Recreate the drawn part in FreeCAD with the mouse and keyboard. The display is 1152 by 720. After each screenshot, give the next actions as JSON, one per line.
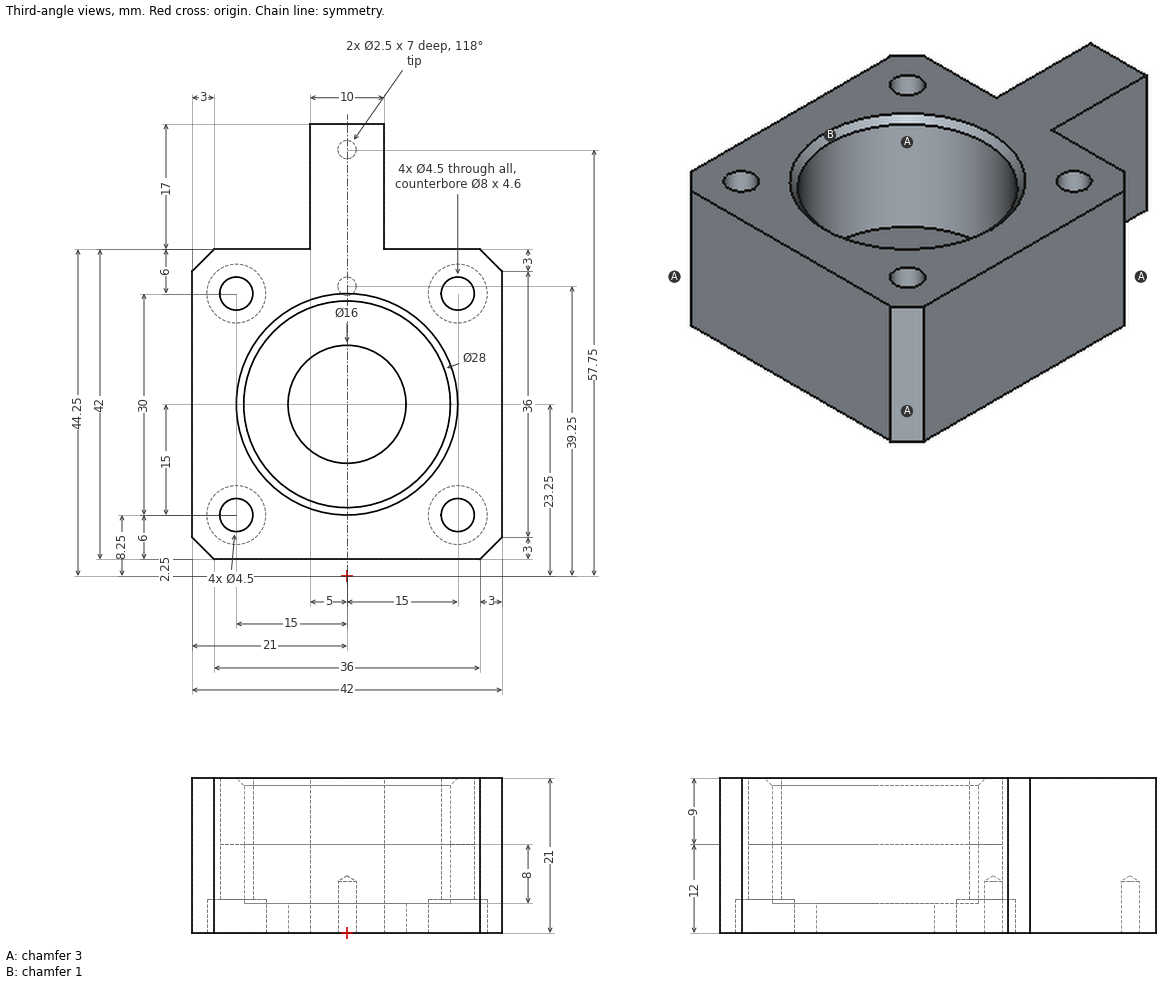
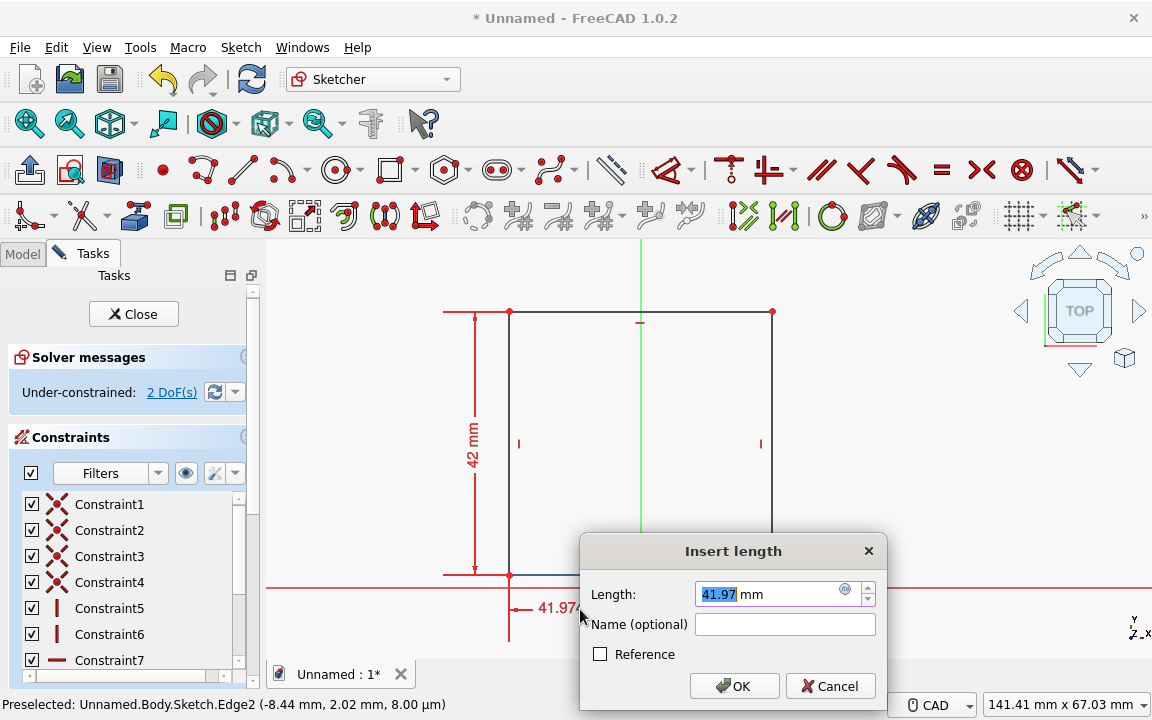
{"action": "type", "text": "42"}
{"action": "key", "text": "Return"}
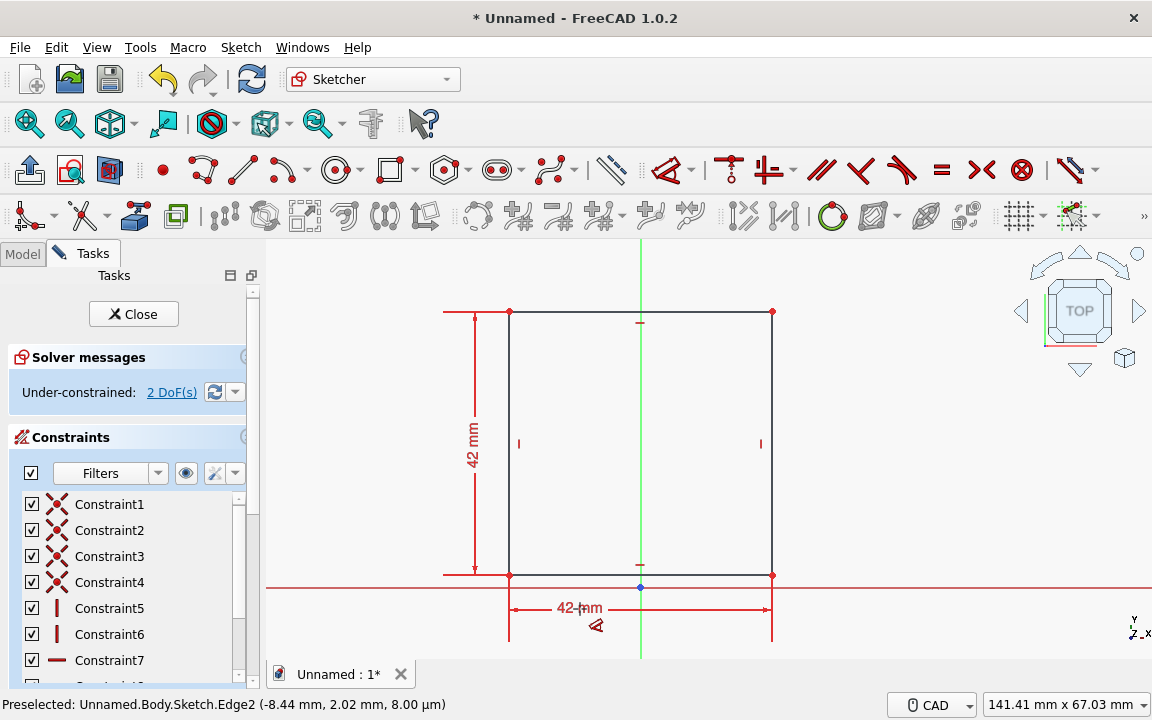
{"action": "left_click", "coordinate": [509, 312]}
{"action": "left_click", "coordinate": [575, 278]}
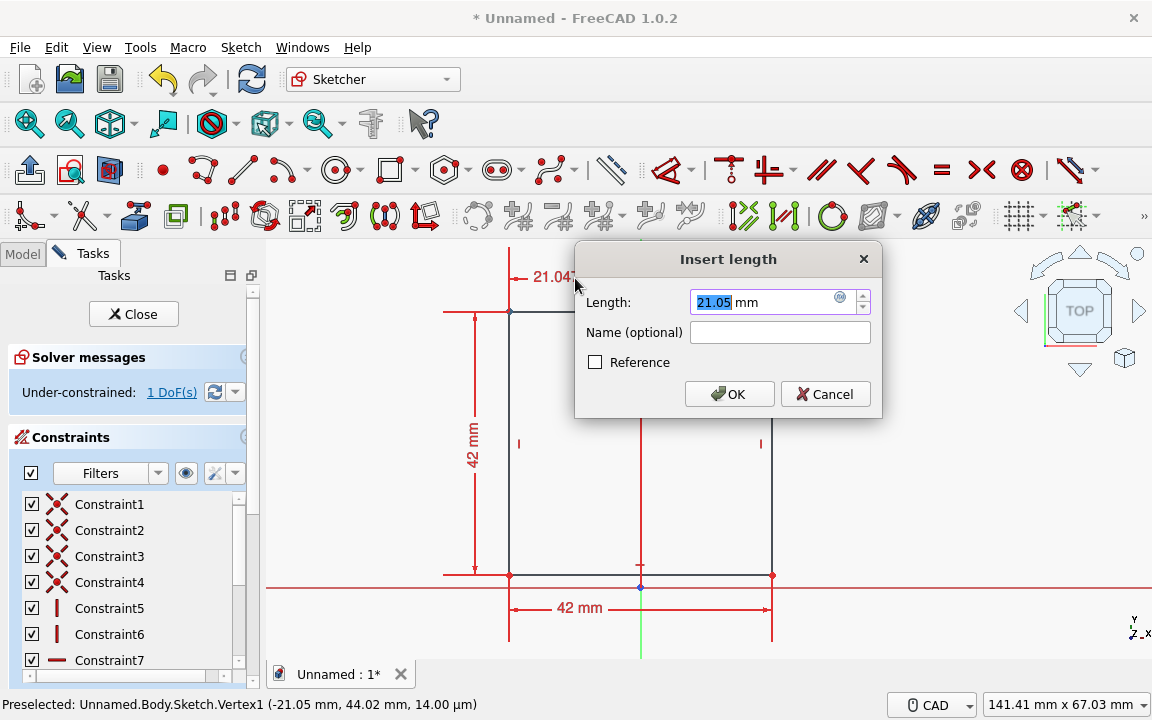
{"action": "type", "text": "21"}
{"action": "key", "text": "Return"}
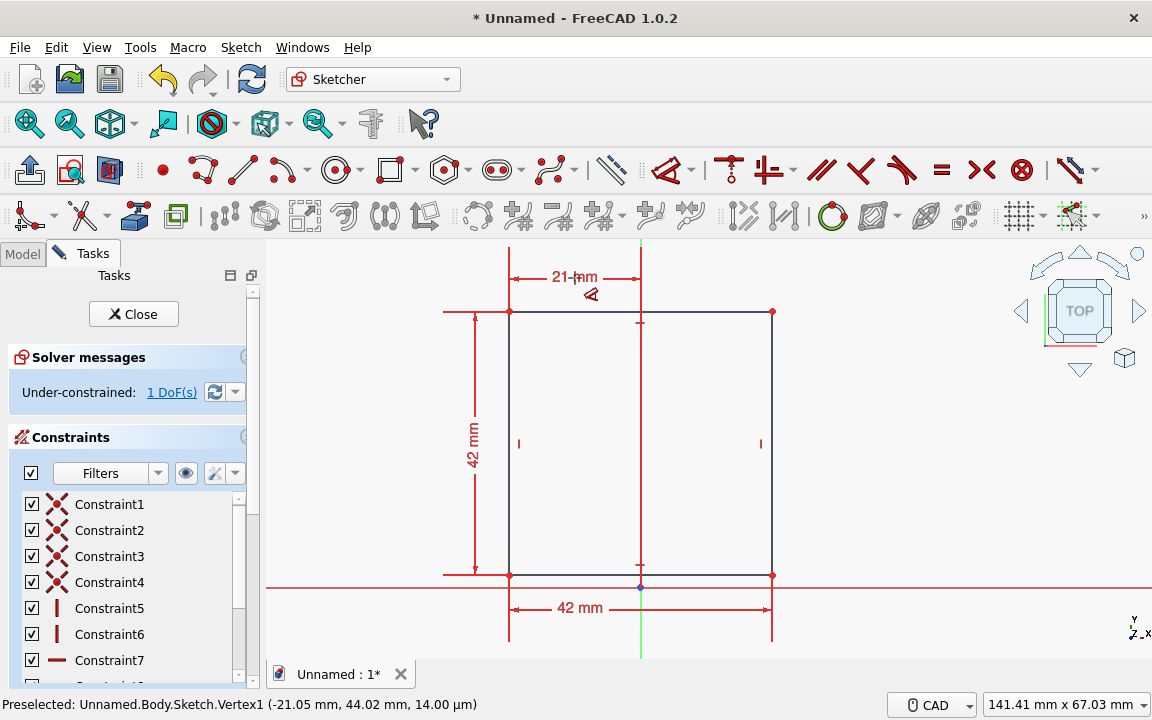
{"action": "scroll", "coordinate": [509, 575], "scroll_direction": "up", "scroll_amount": 6}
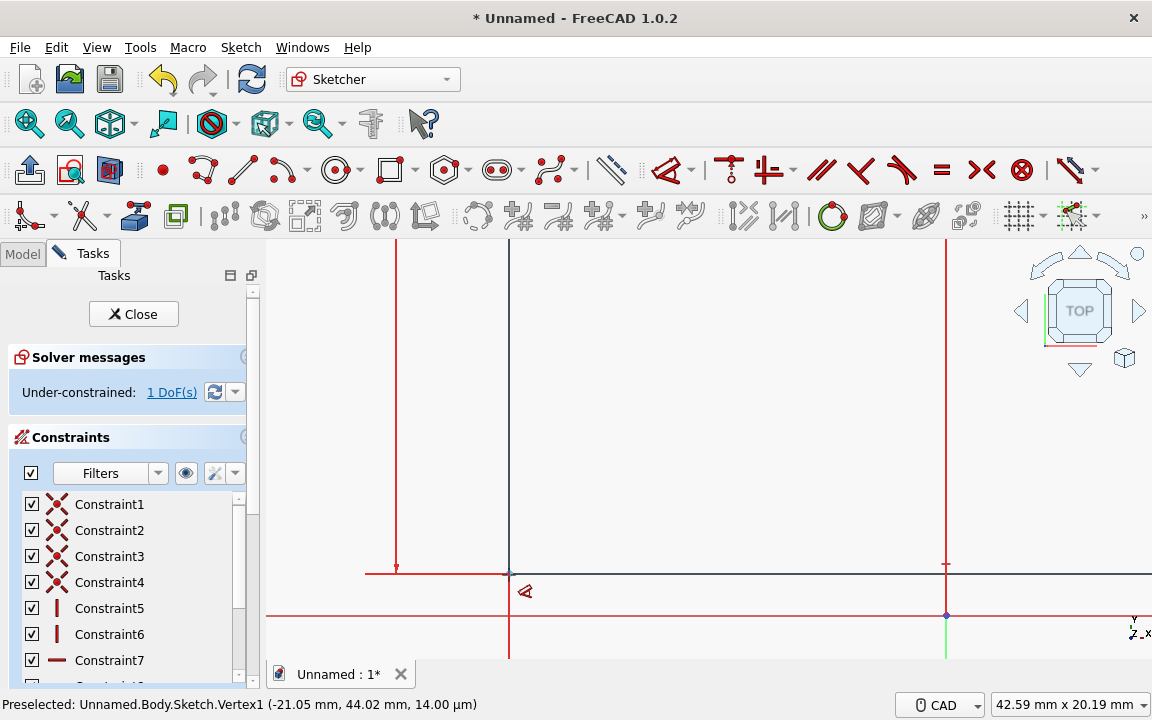
{"action": "left_click", "coordinate": [509, 574]}
{"action": "left_click", "coordinate": [475, 595]}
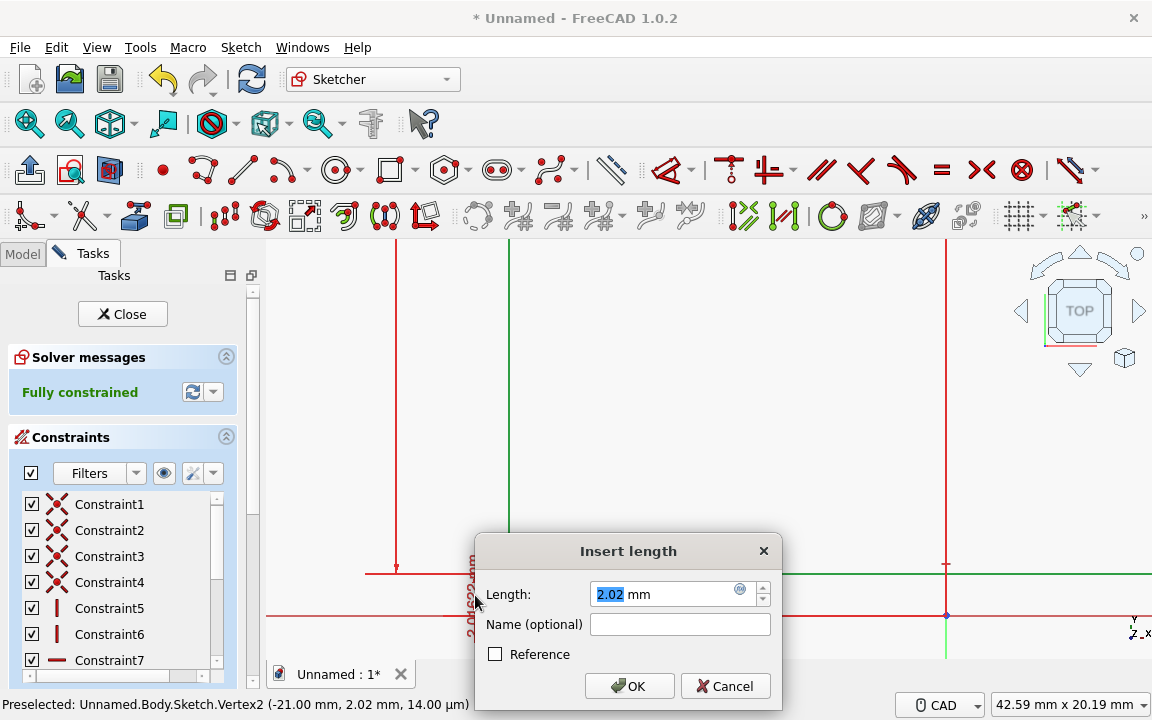
{"action": "type", "text": "2.25"}
{"action": "key", "text": "Return"}
{"action": "key", "text": "Escape"}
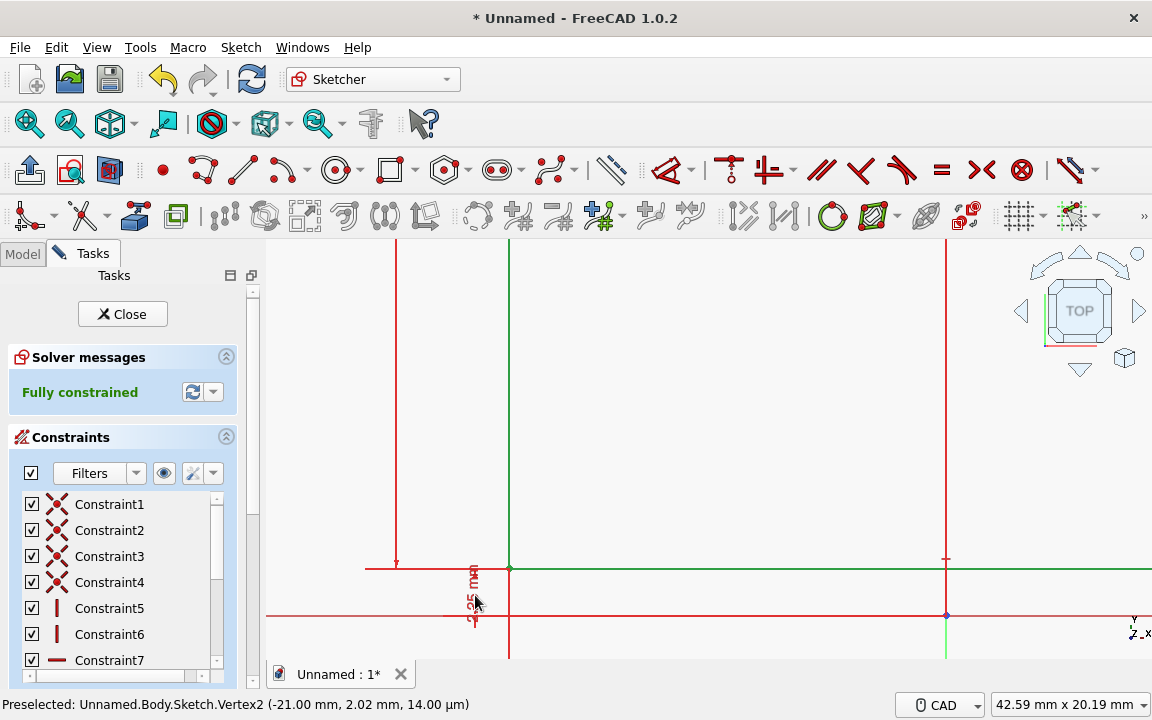
{"action": "left_click", "coordinate": [123, 314]}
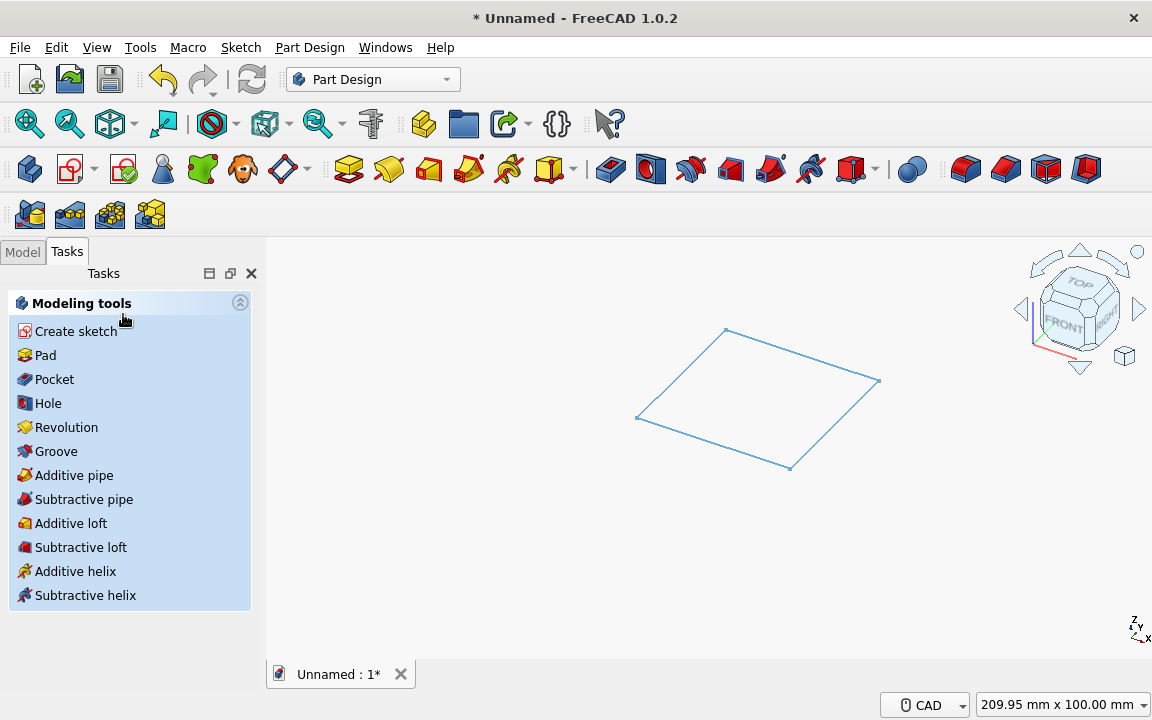
{"action": "left_click", "coordinate": [350, 170]}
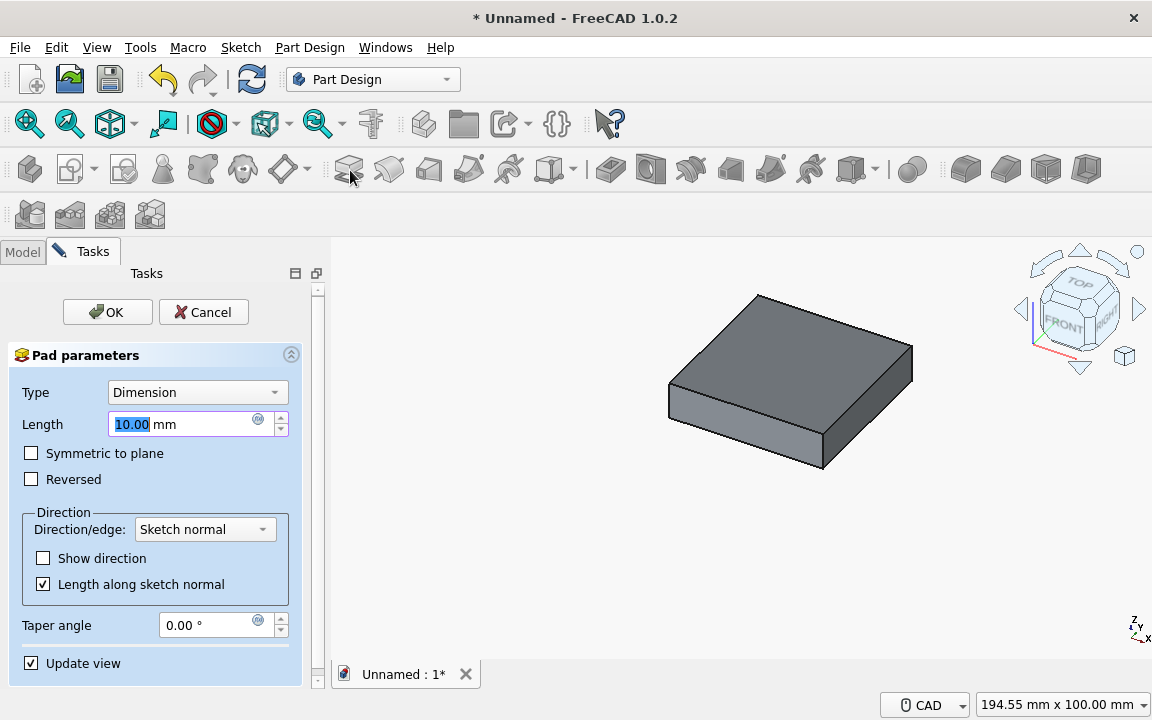
{"action": "type", "text": "12"}
{"action": "key", "text": "Tab"}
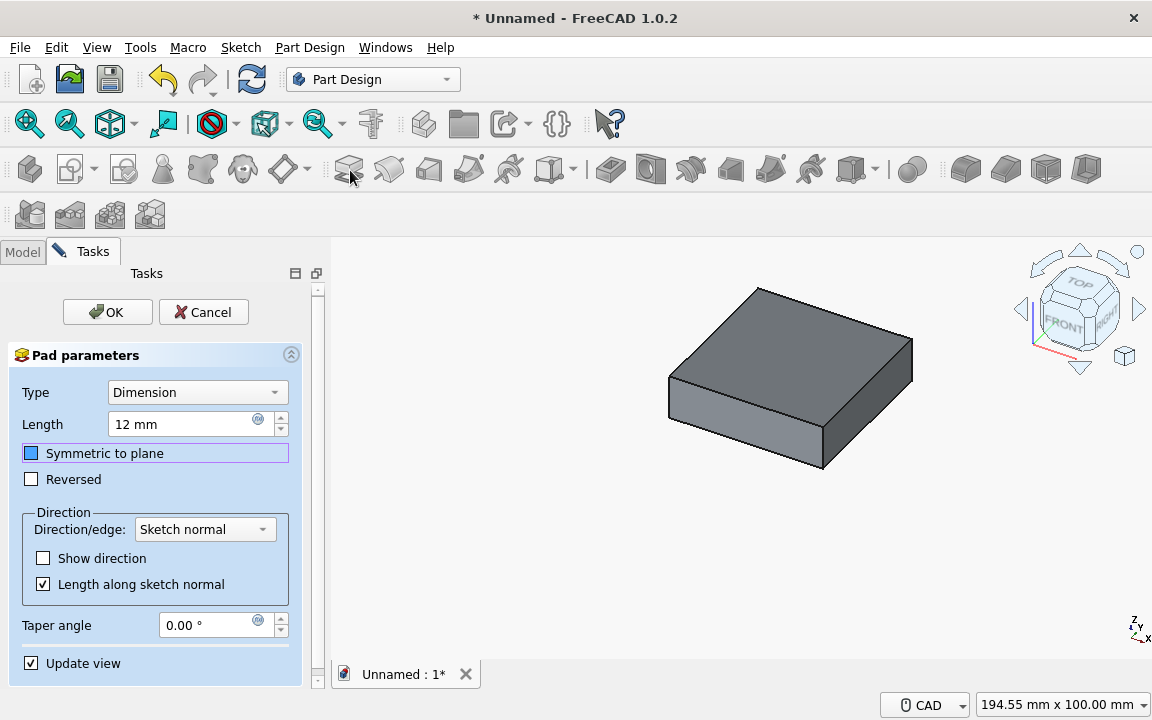
{"action": "left_click", "coordinate": [108, 312]}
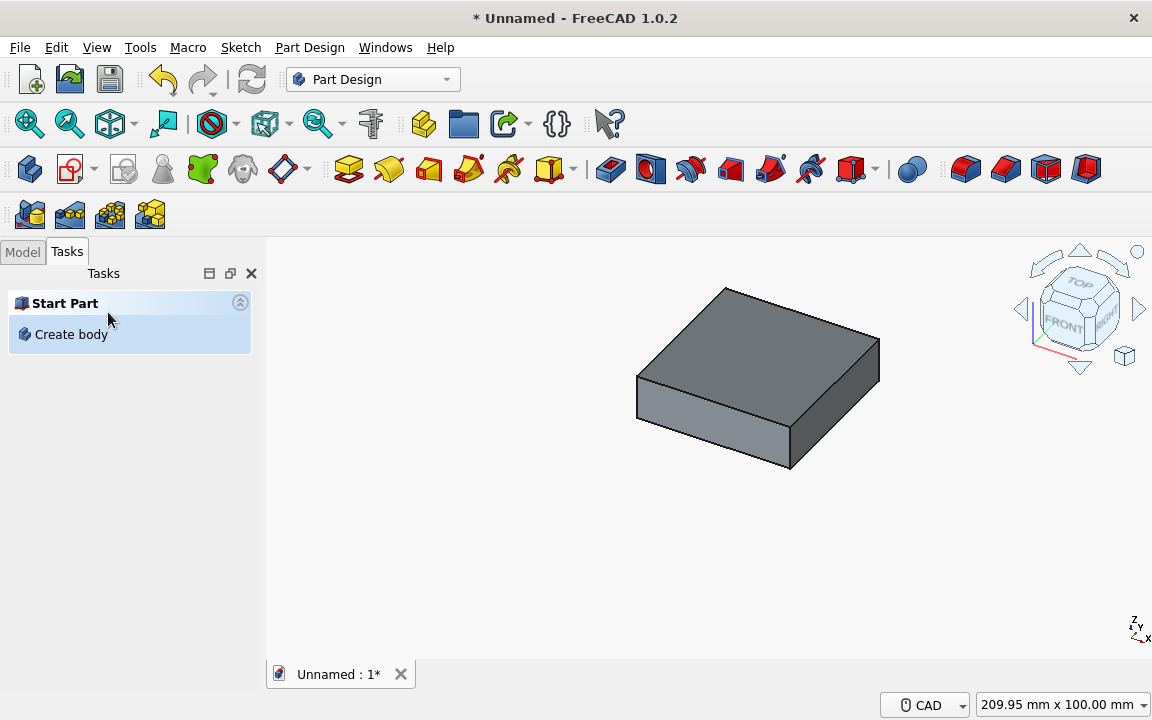
{"action": "left_click", "coordinate": [30, 124]}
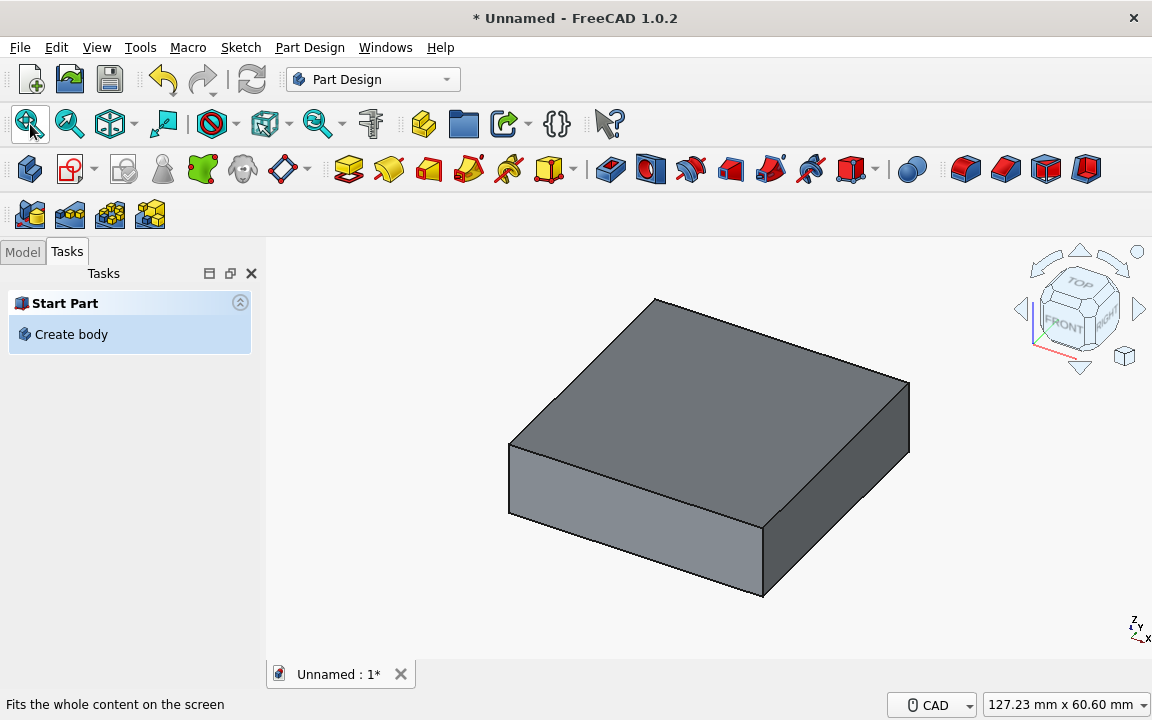
{"action": "left_click", "coordinate": [709, 413]}